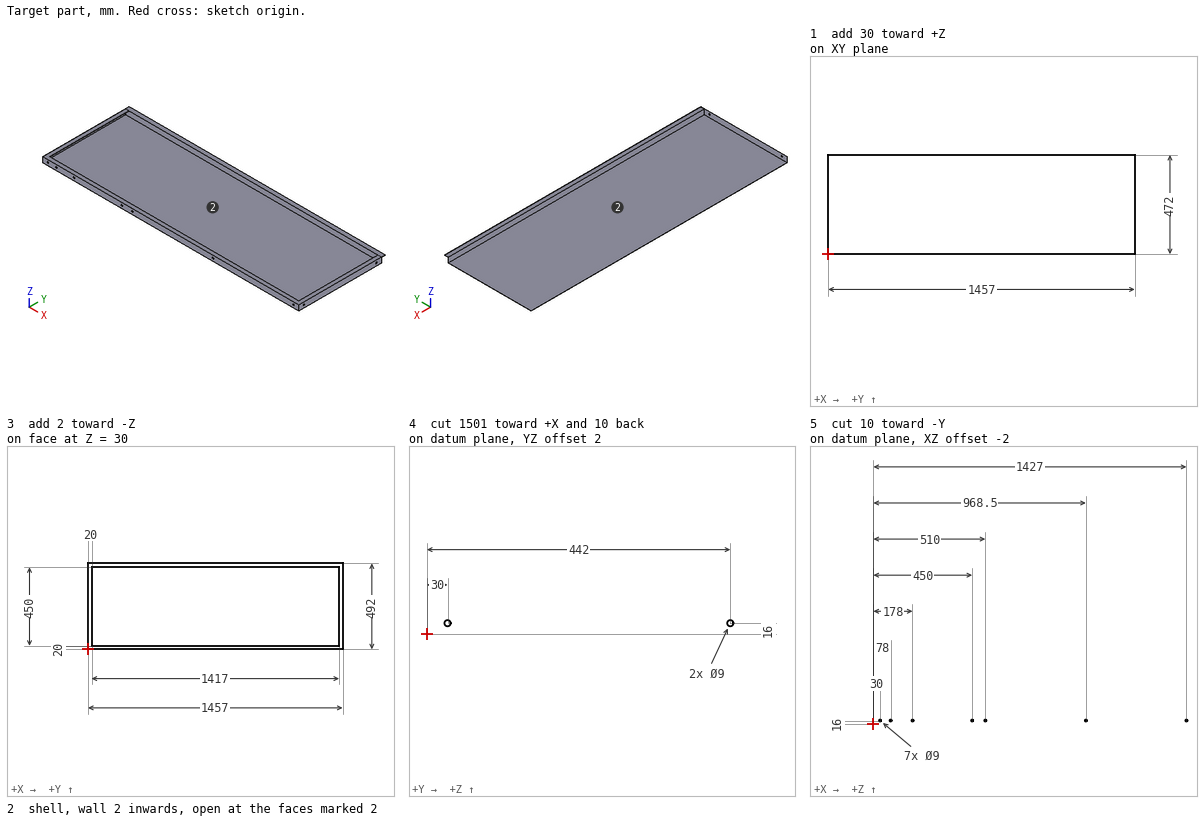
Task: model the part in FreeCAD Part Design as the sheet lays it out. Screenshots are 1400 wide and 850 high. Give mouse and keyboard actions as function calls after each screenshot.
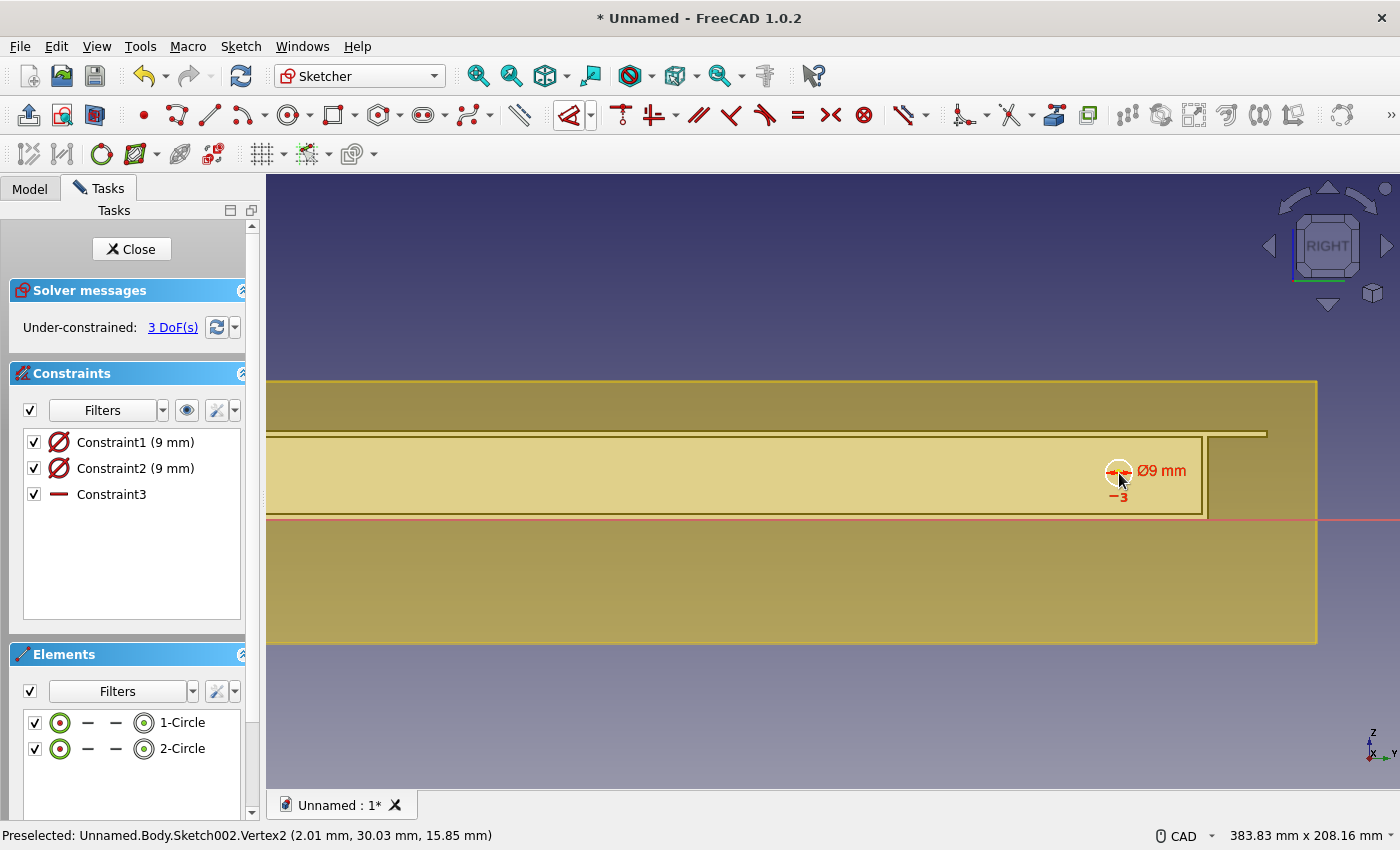
click(1119, 473)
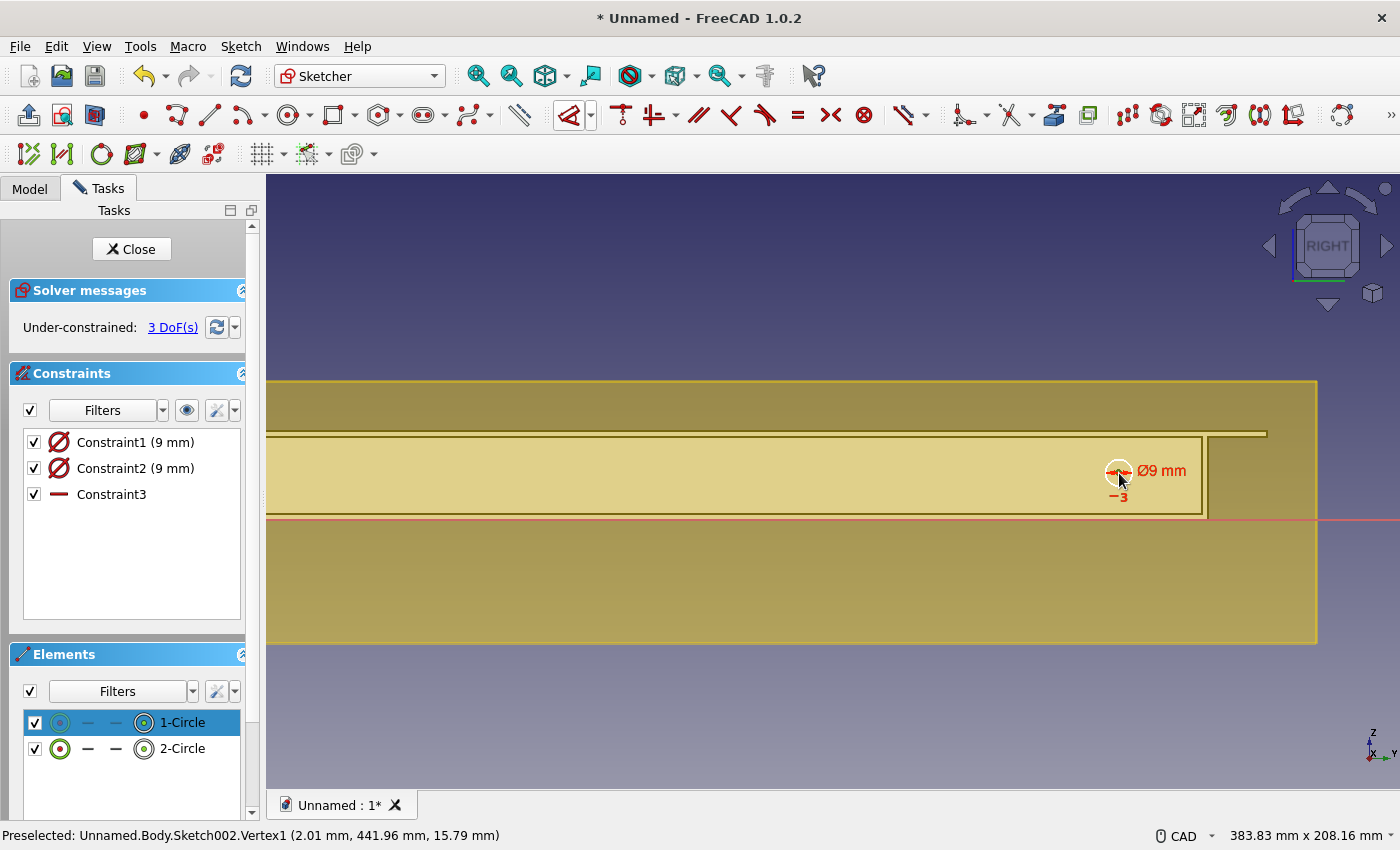
key(i)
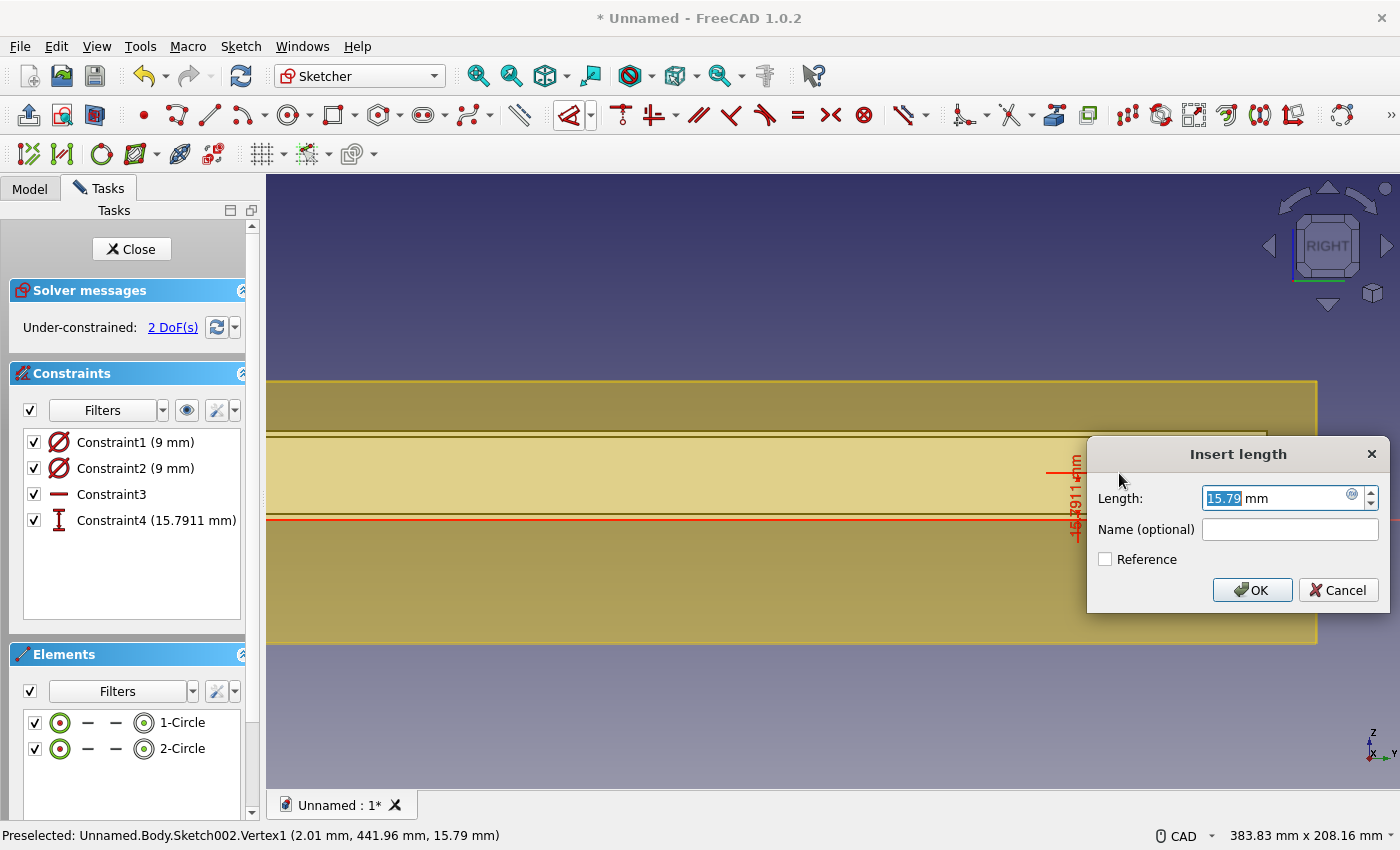
text(16)
key(Return)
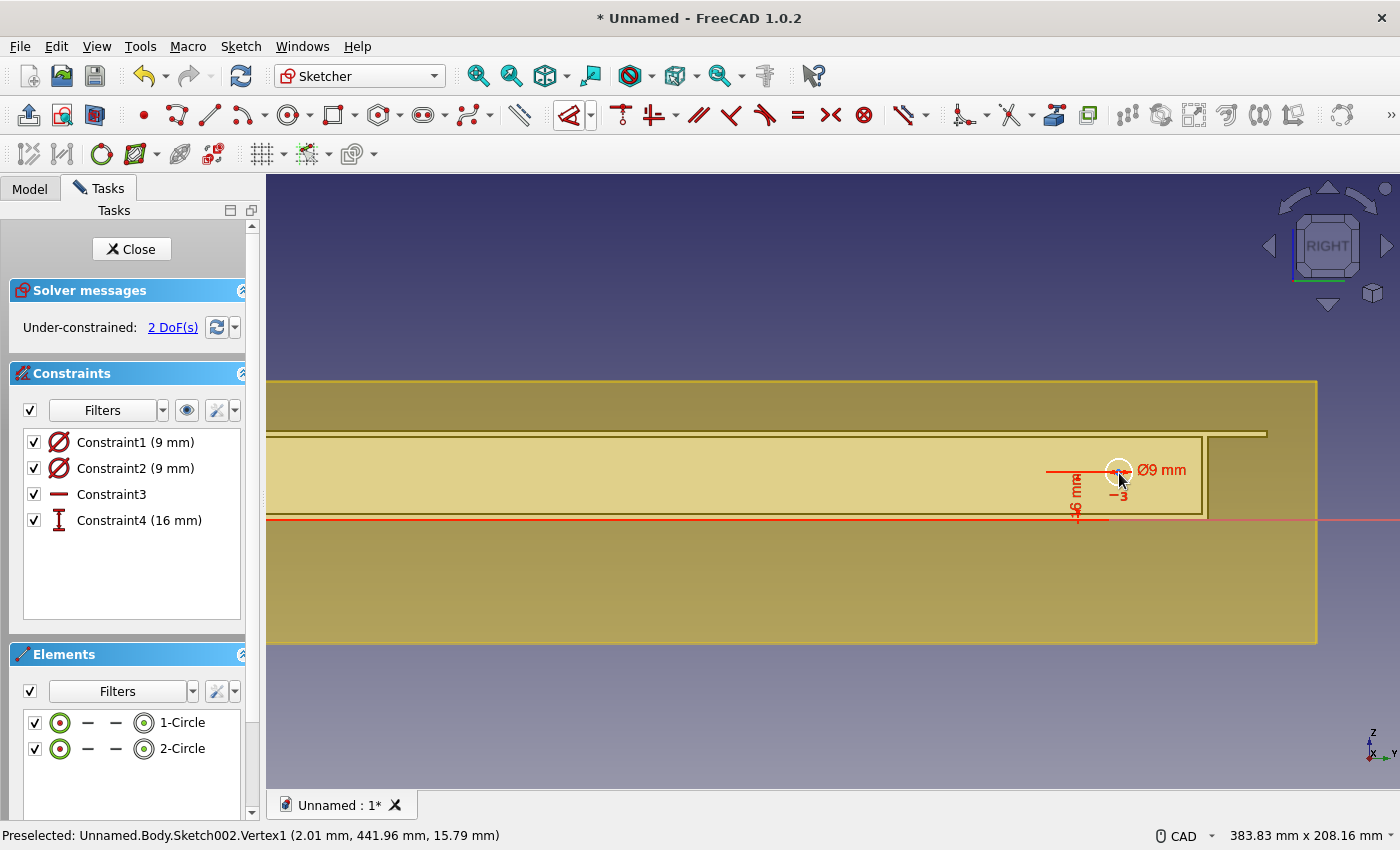
scroll(1119, 472, down, 3)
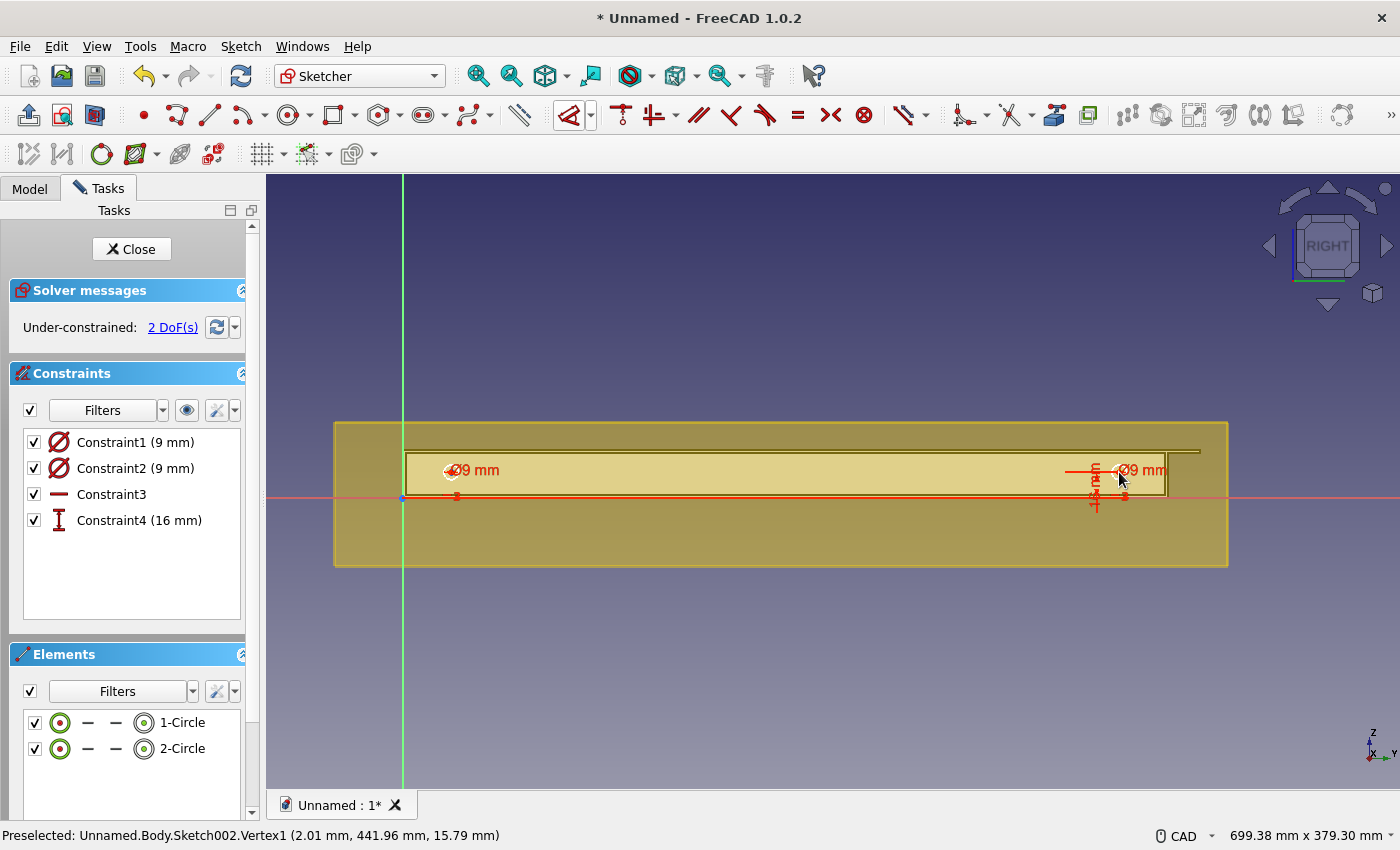
click(451, 472)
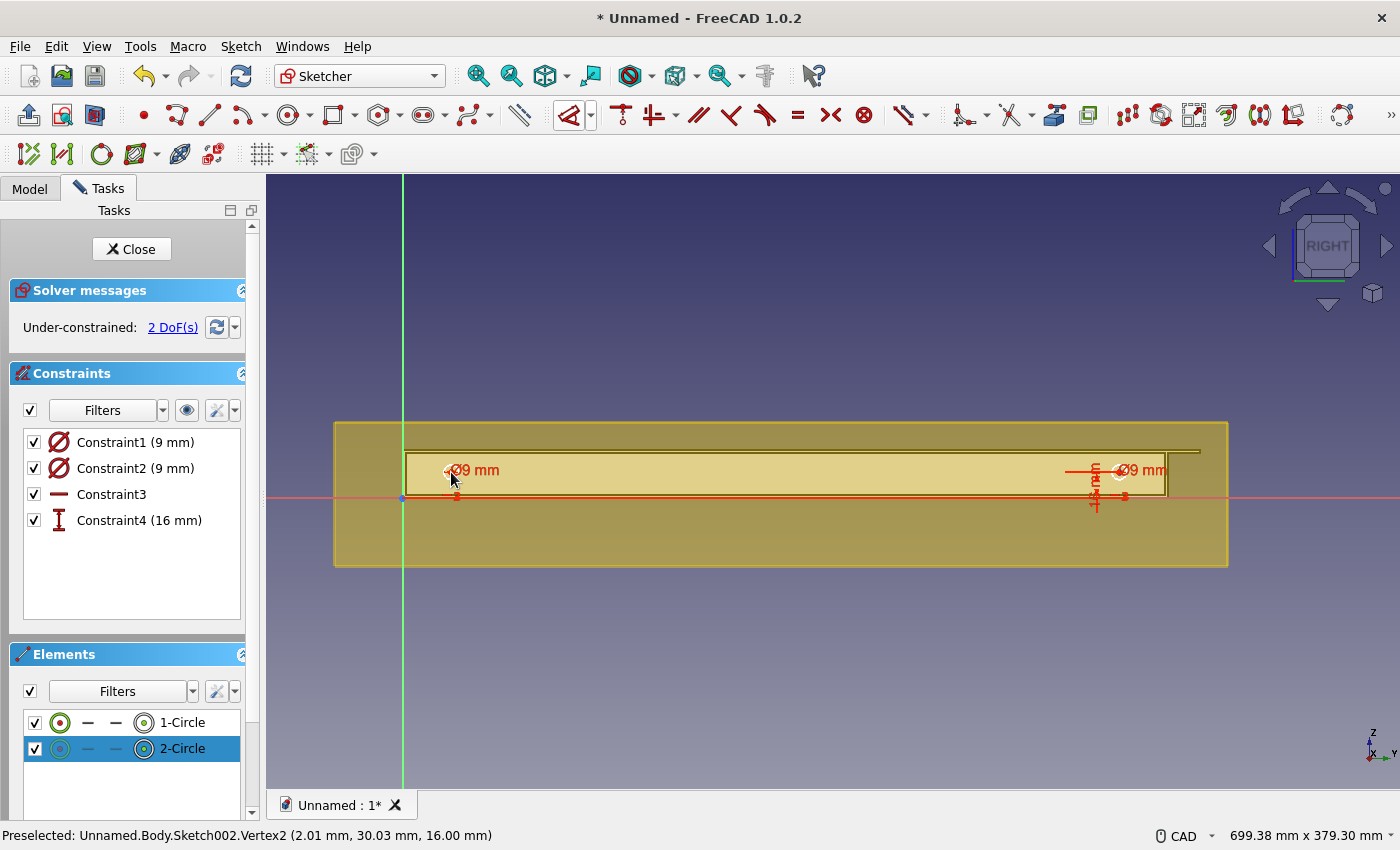
click(590, 116)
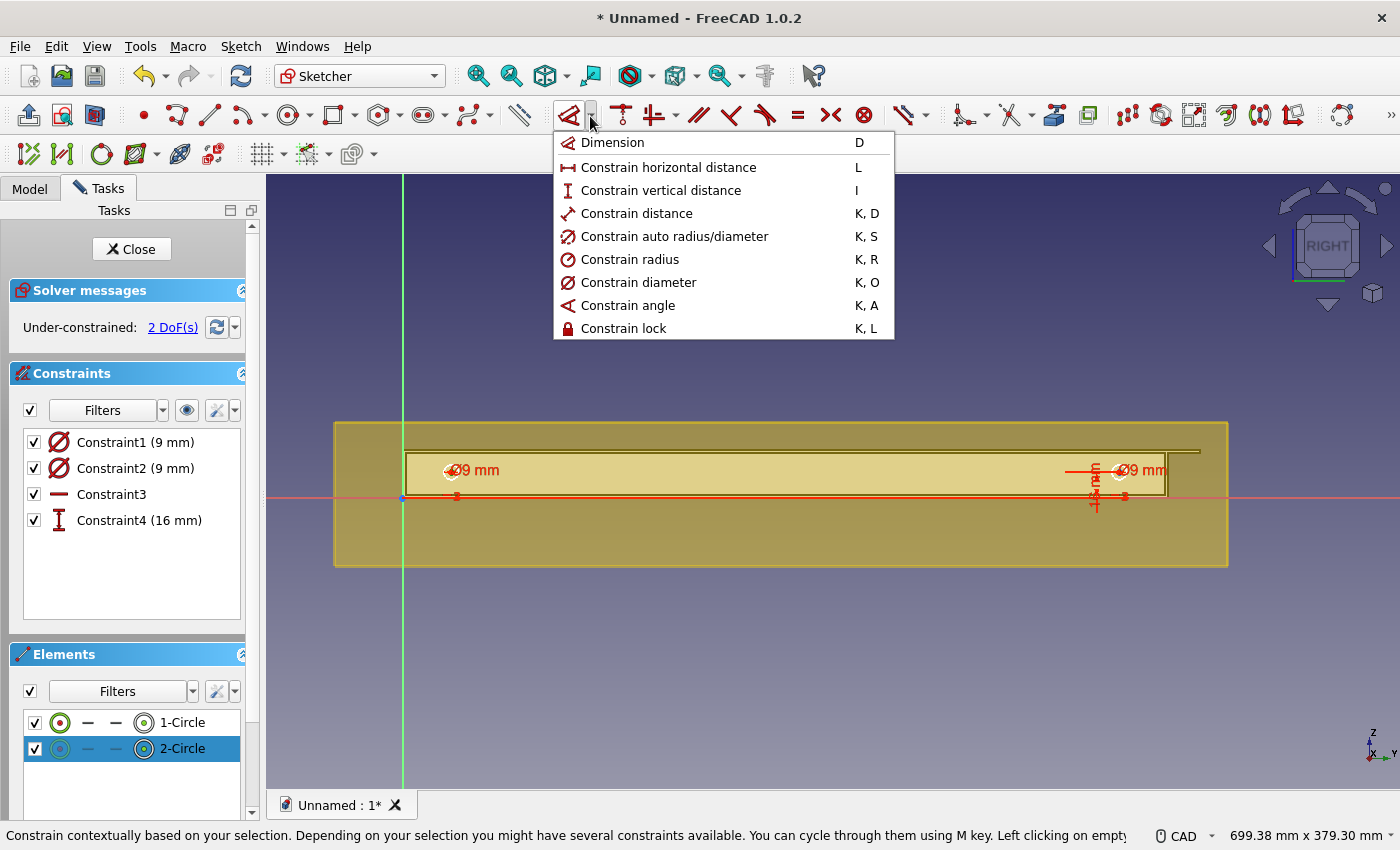
click(724, 168)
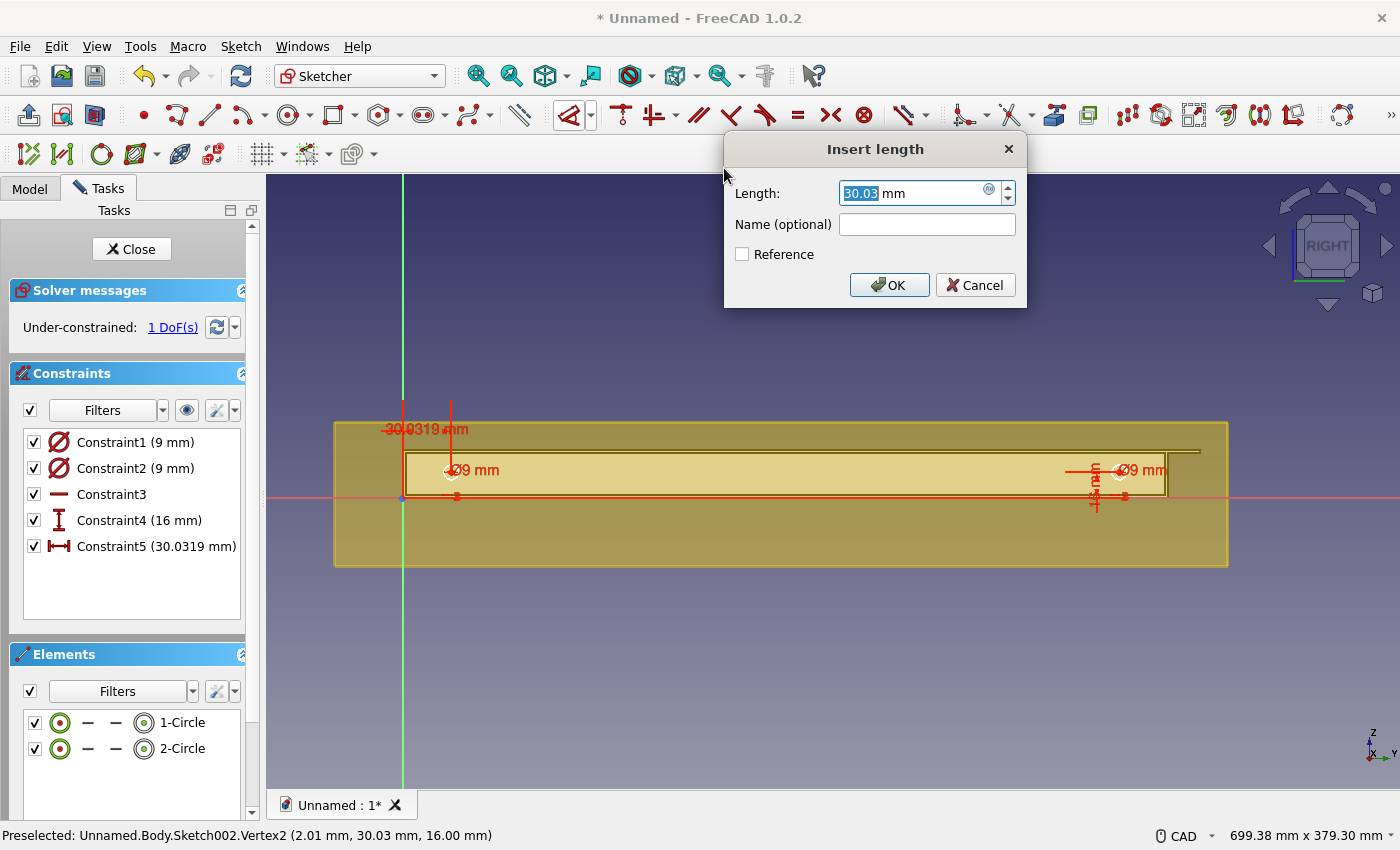
text(30)
key(Return)